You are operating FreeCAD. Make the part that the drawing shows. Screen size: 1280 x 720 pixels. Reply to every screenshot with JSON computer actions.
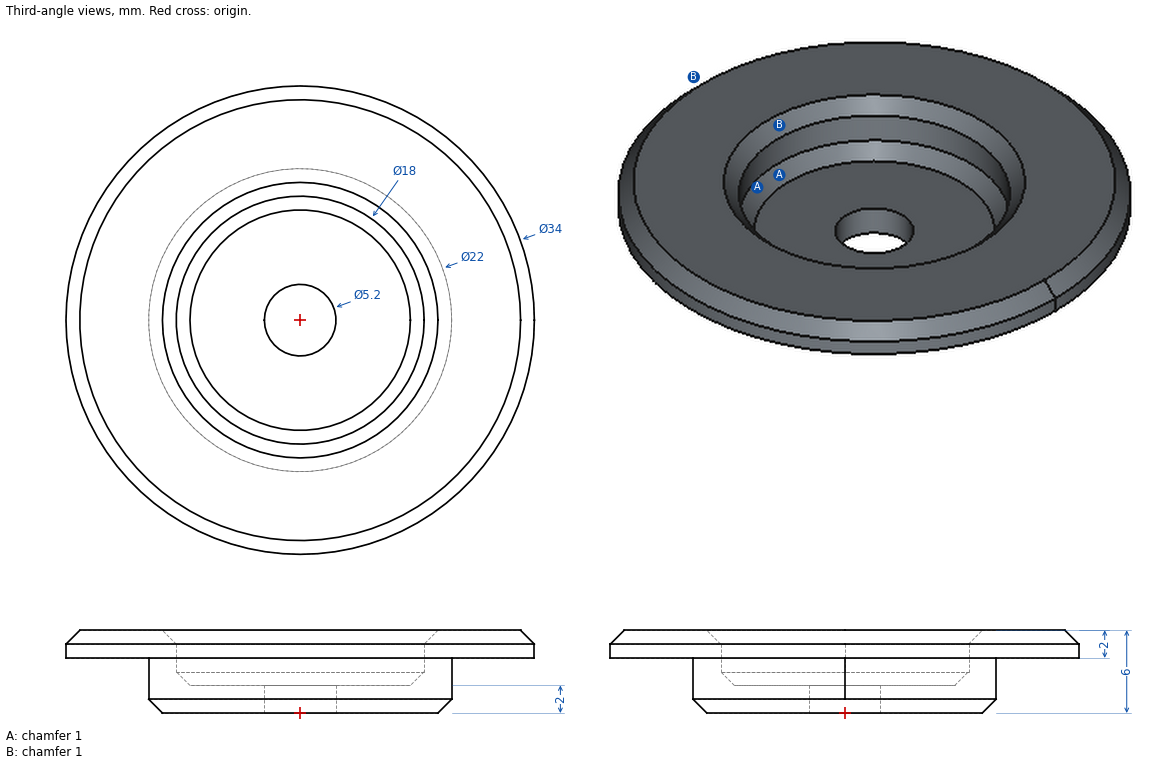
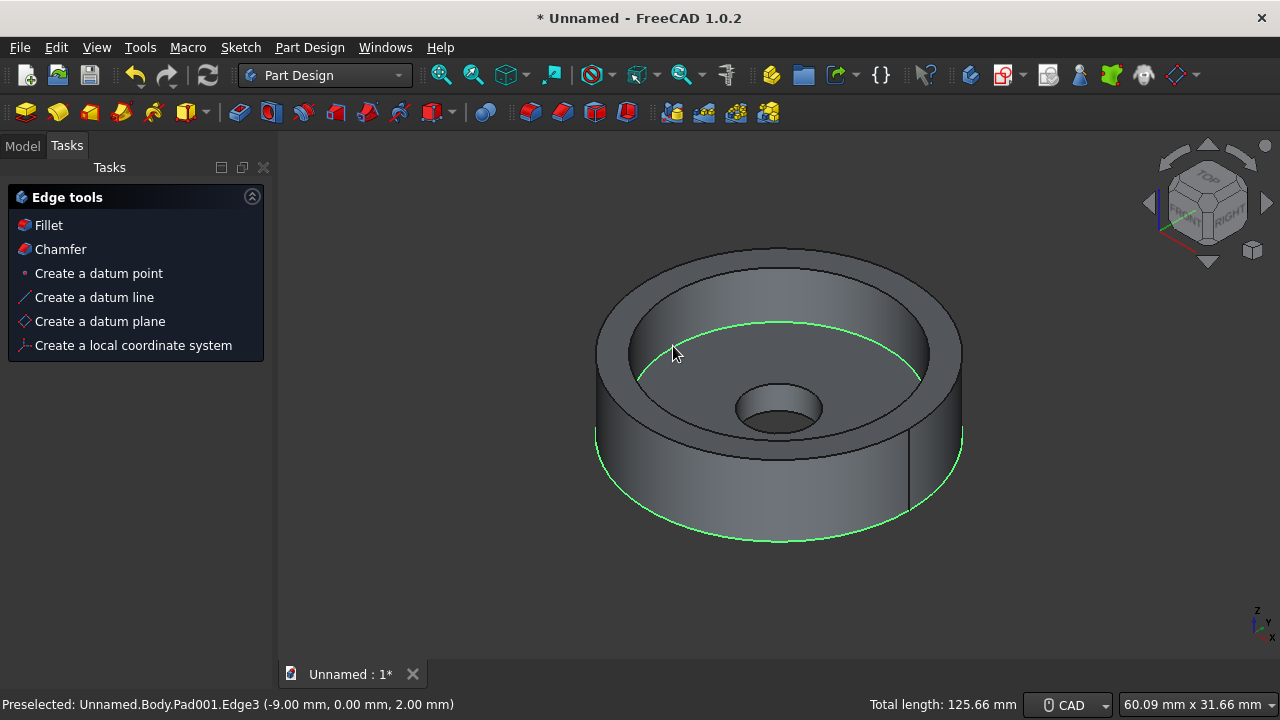
{"action": "left_click", "coordinate": [564, 112]}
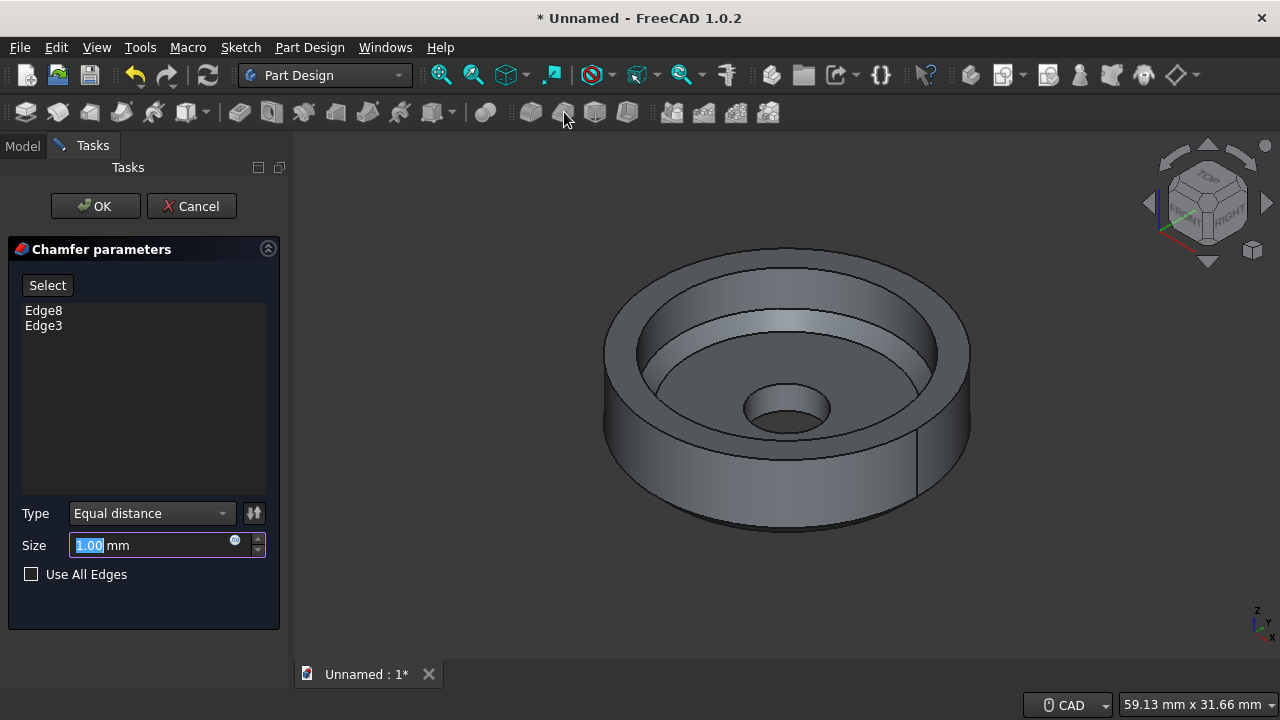
{"action": "type", "text": "1"}
{"action": "key", "text": "Tab"}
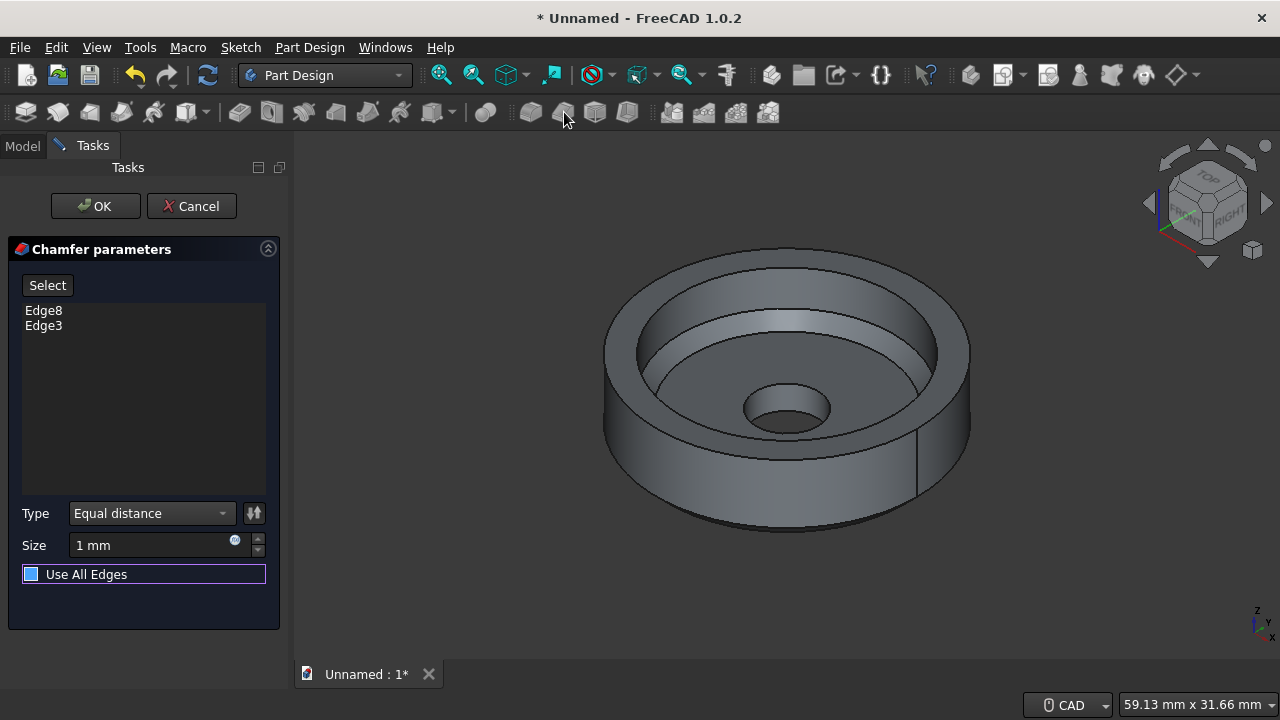
{"action": "left_click", "coordinate": [96, 206]}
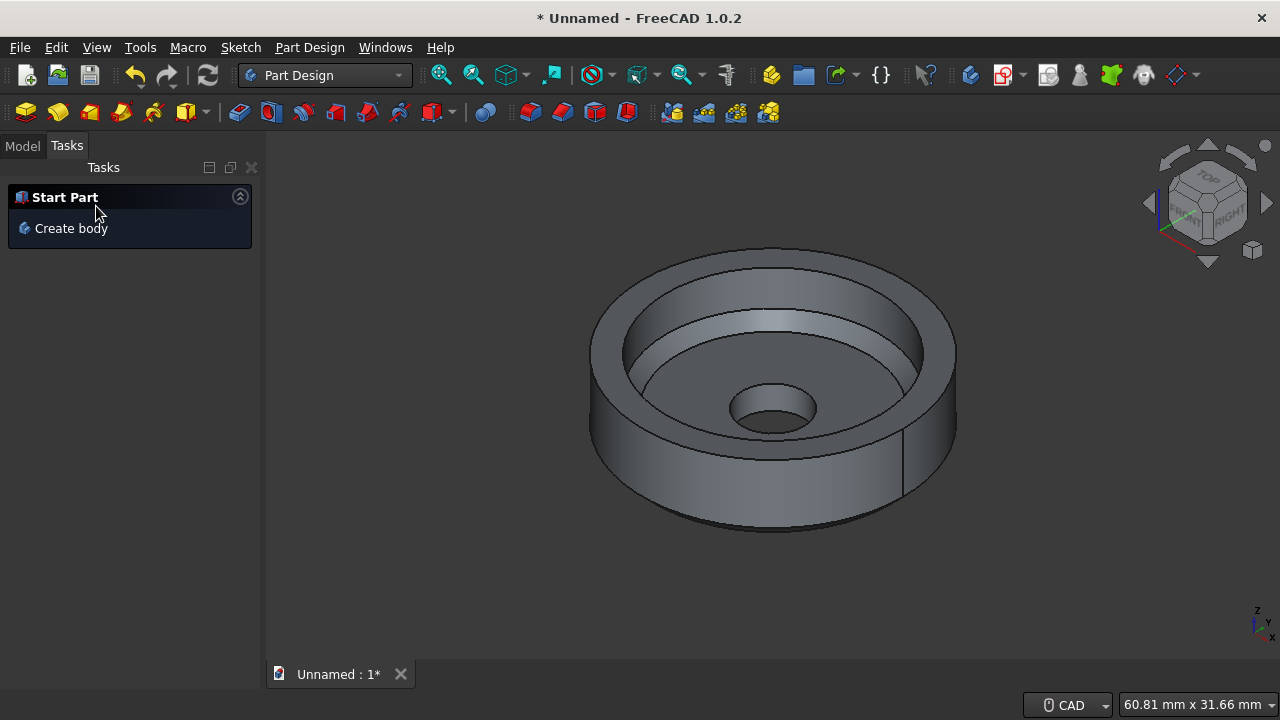
{"action": "left_click", "coordinate": [23, 145]}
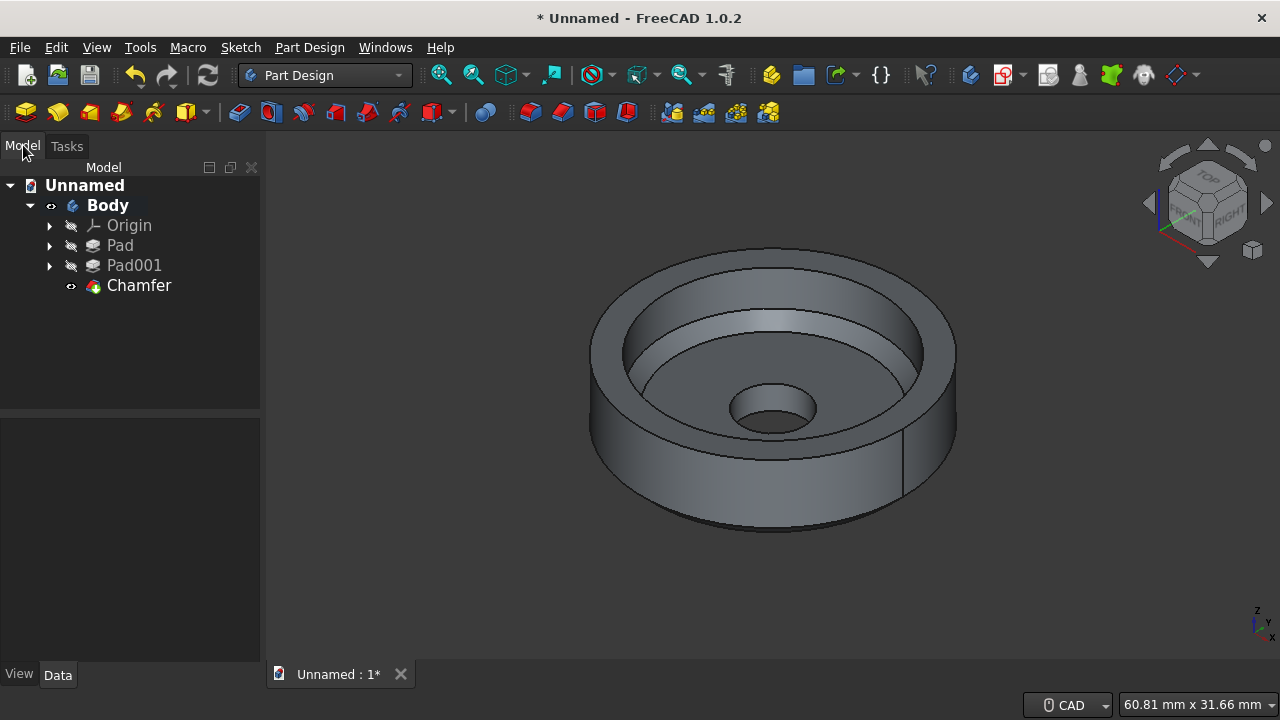
{"action": "left_click", "coordinate": [50, 226]}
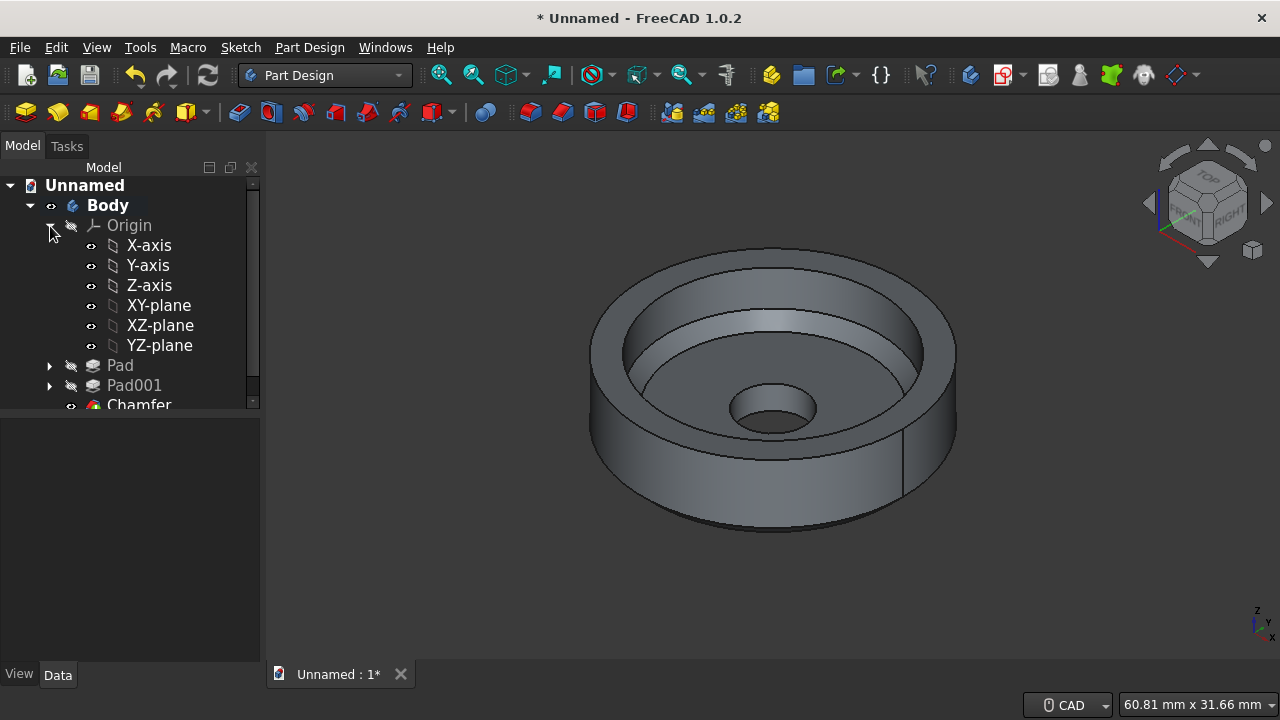
{"action": "left_click", "coordinate": [136, 306]}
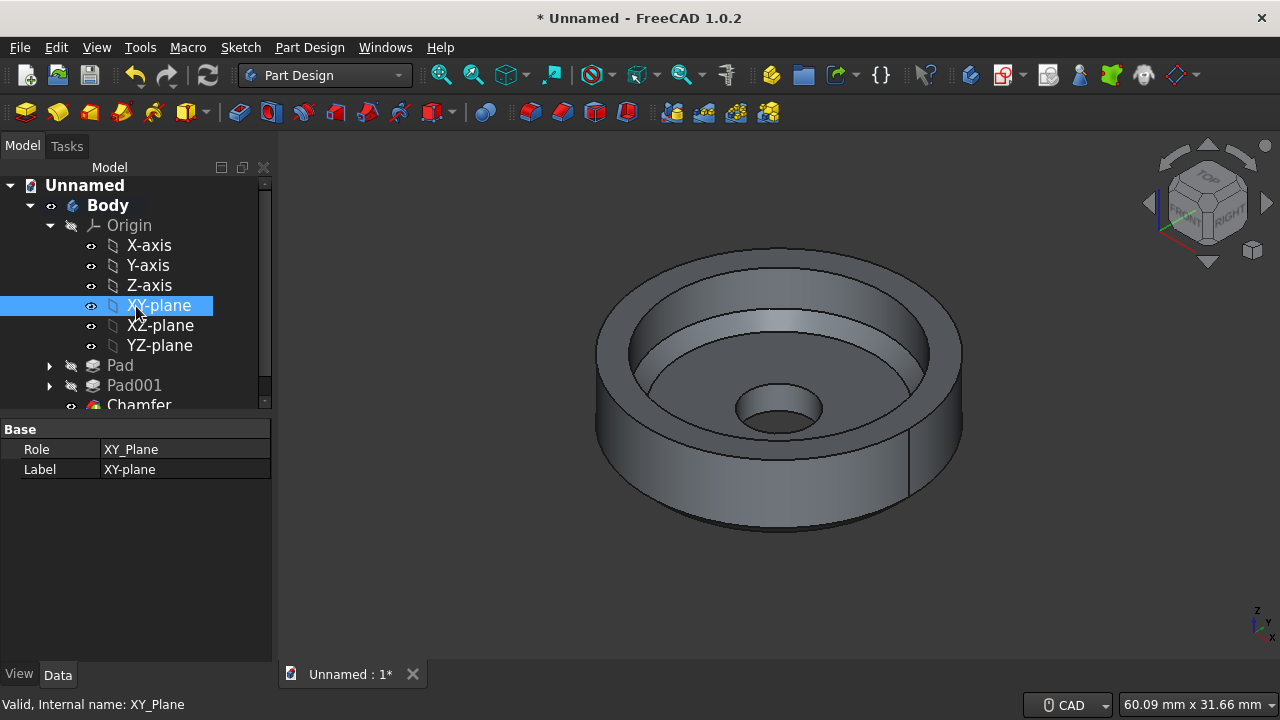
{"action": "left_click", "coordinate": [1176, 76]}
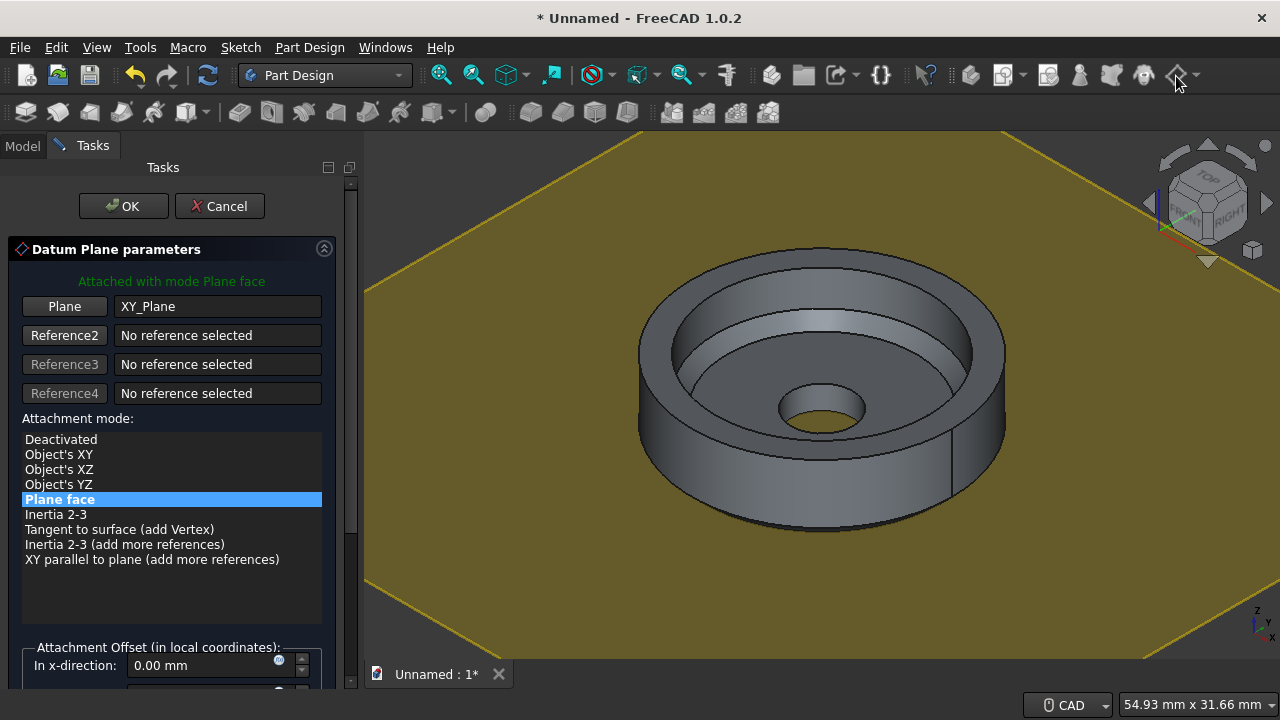
{"action": "scroll", "coordinate": [351, 432], "scroll_direction": "down", "scroll_amount": 2}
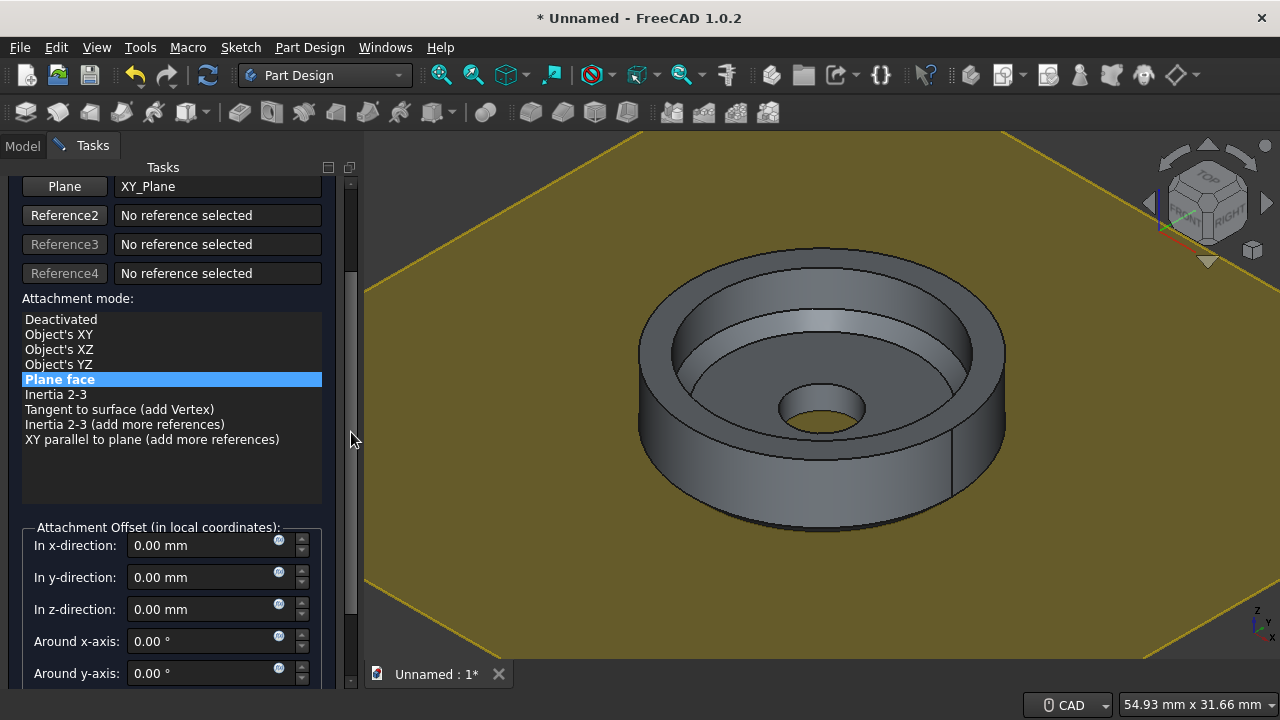
{"action": "triple_click", "coordinate": [210, 609]}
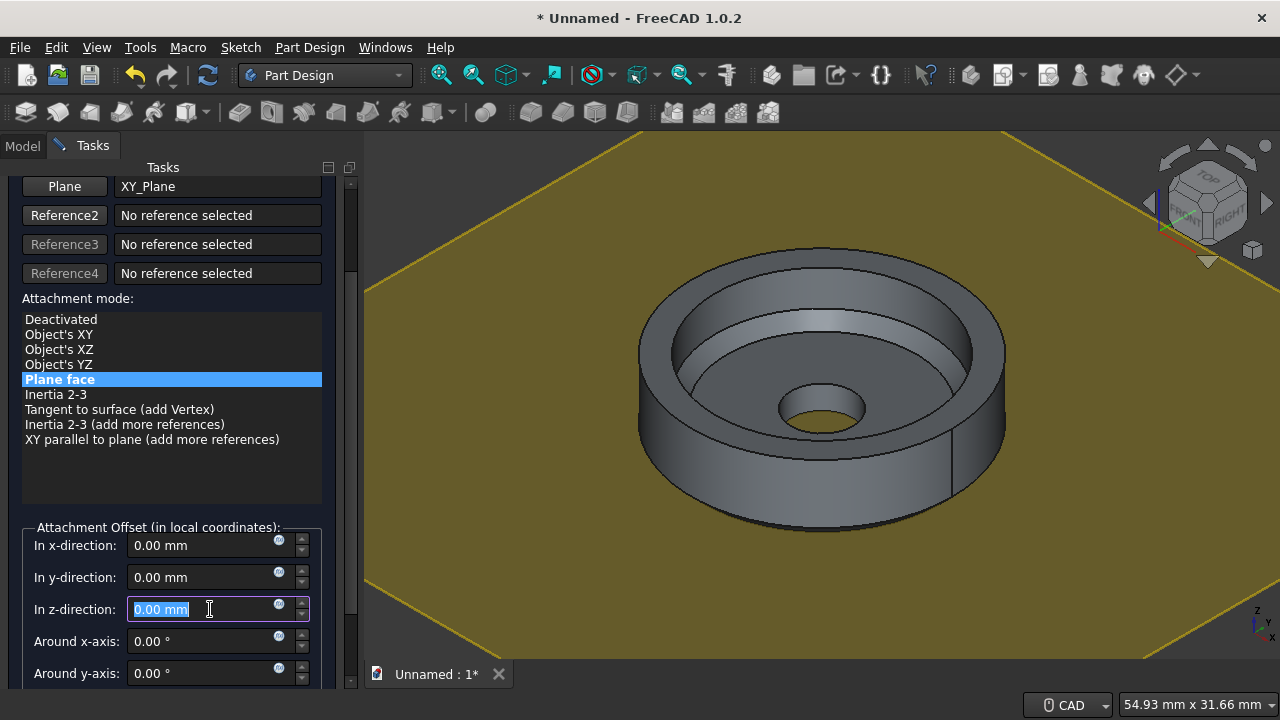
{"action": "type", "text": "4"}
{"action": "key", "text": "Tab"}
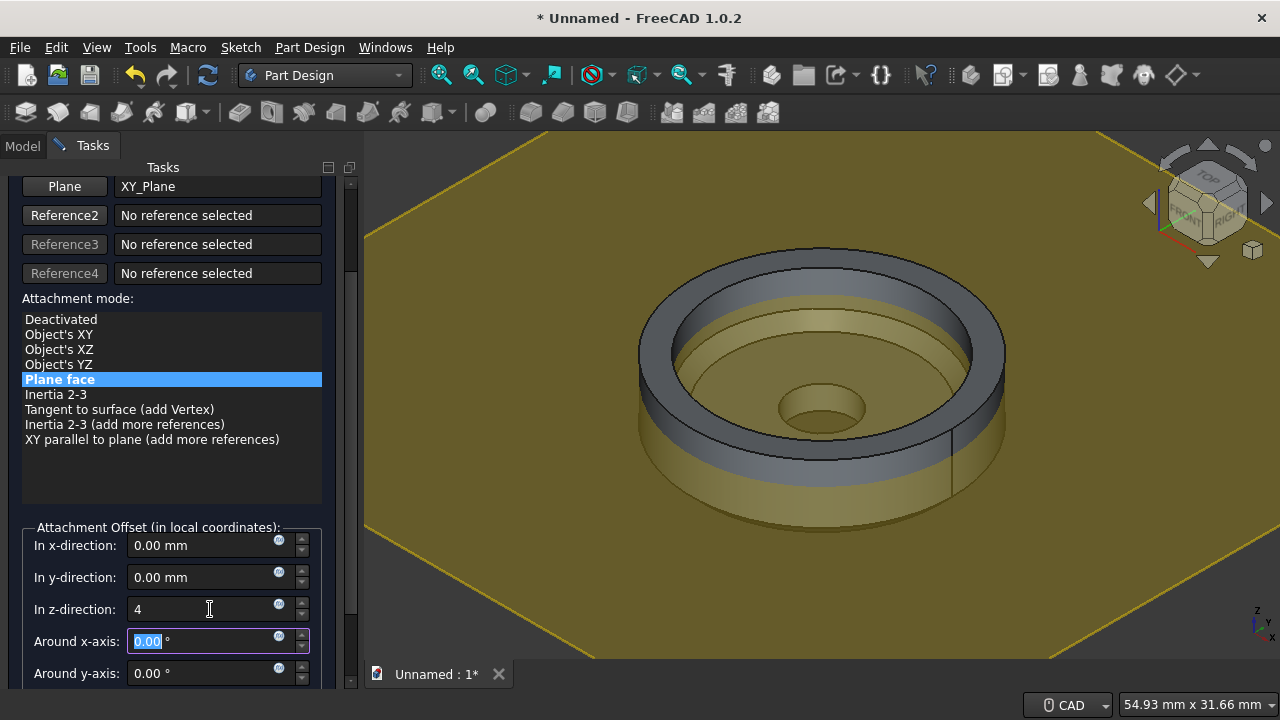
{"action": "scroll", "coordinate": [351, 432], "scroll_direction": "up", "scroll_amount": 3}